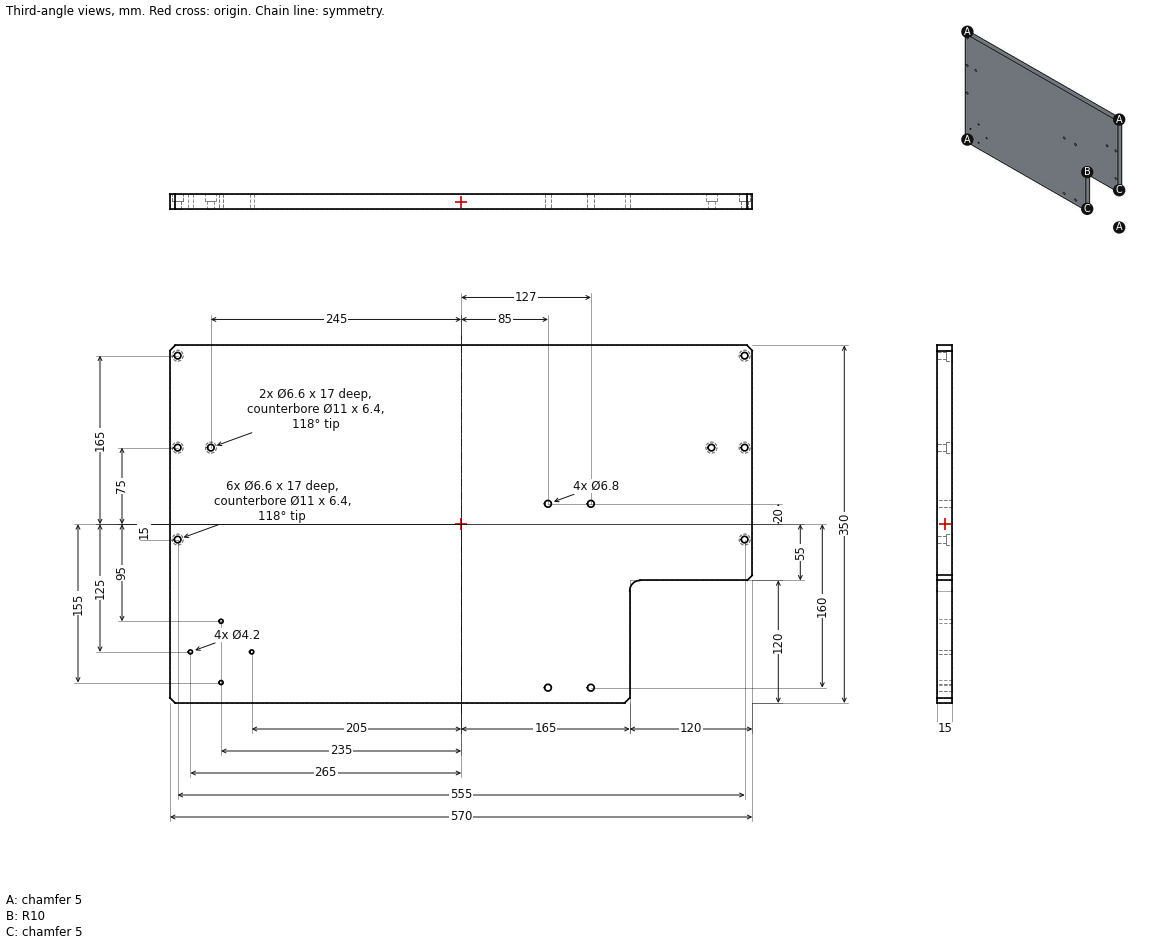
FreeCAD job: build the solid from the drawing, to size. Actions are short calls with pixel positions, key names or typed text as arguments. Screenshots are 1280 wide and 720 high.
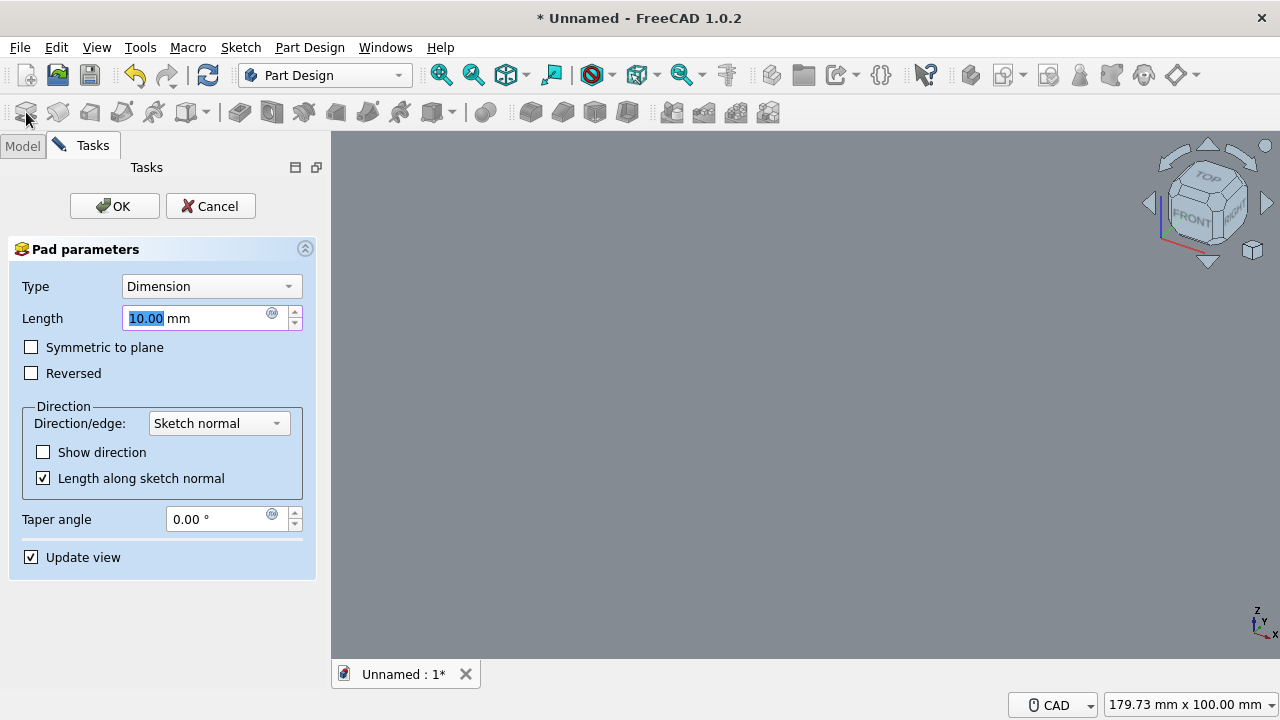
text(15)
key(Tab)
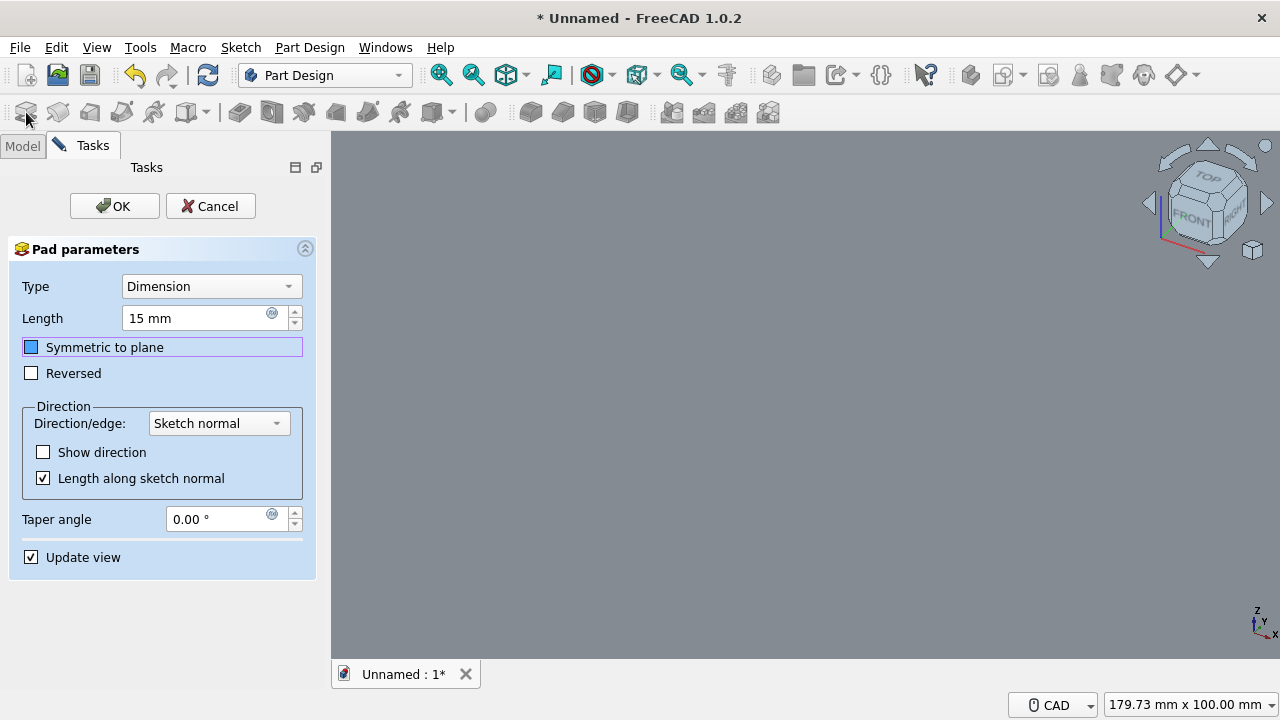
click(30, 347)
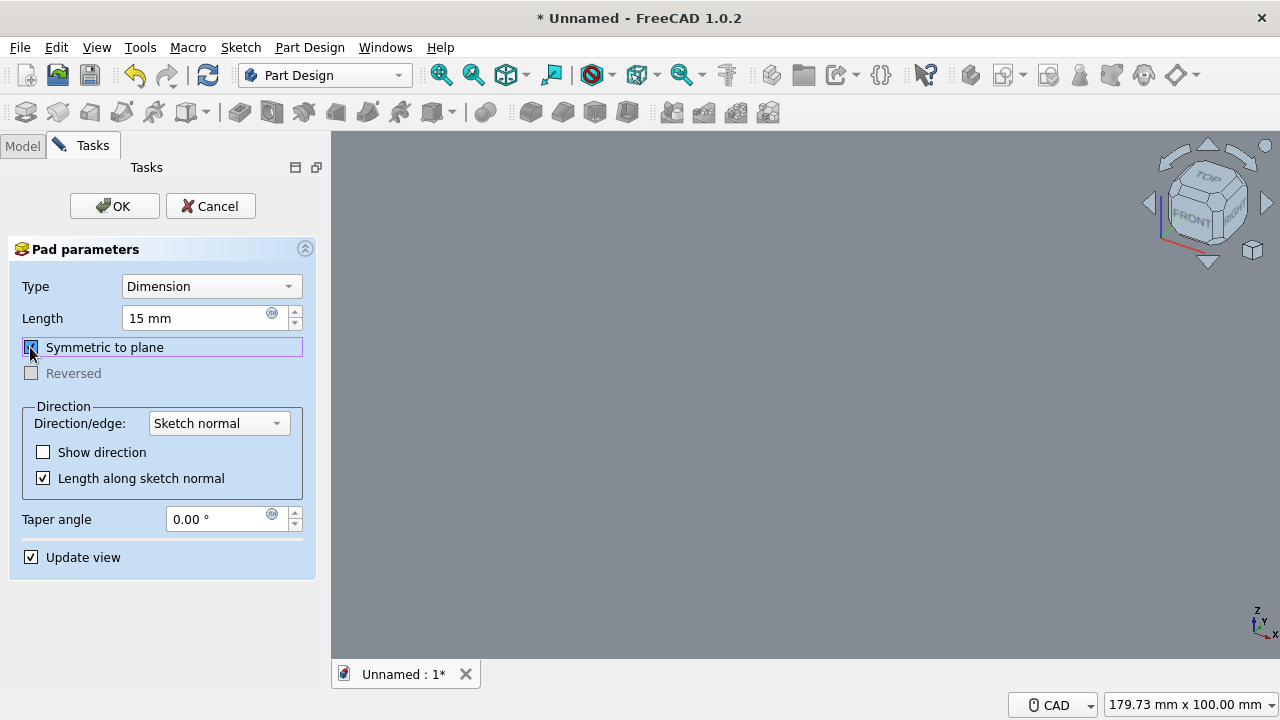
click(115, 206)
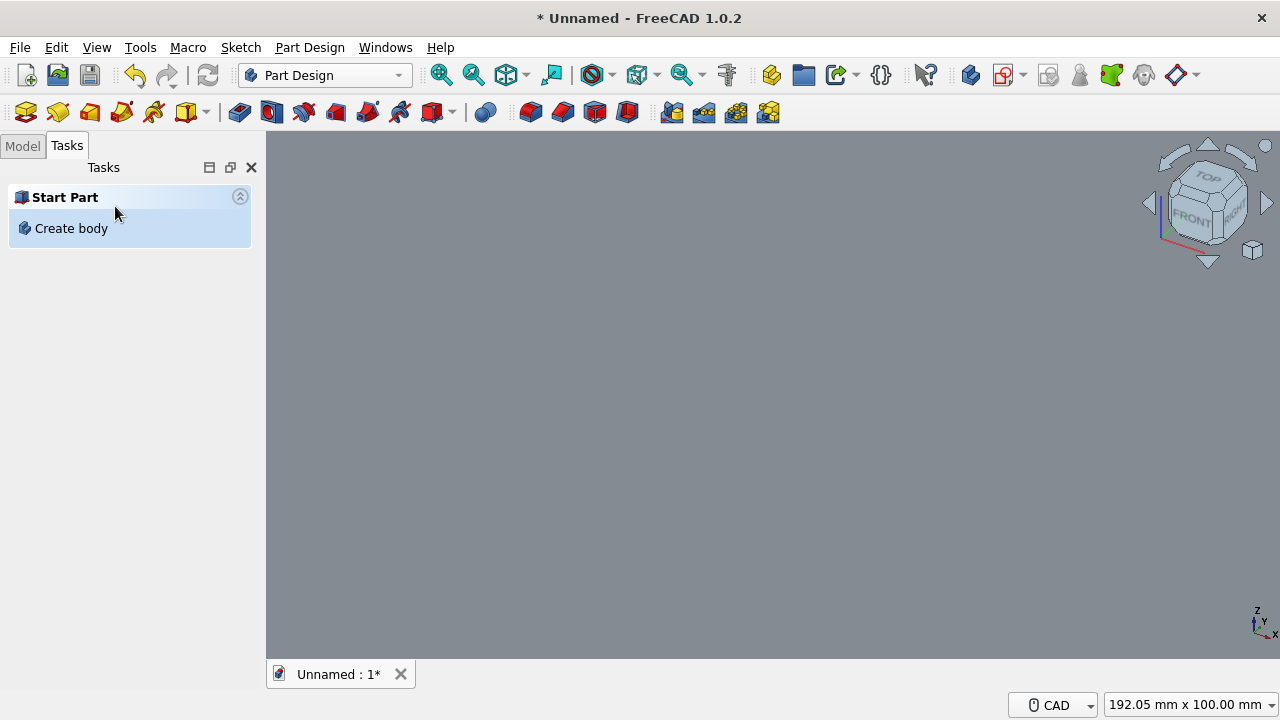
click(442, 76)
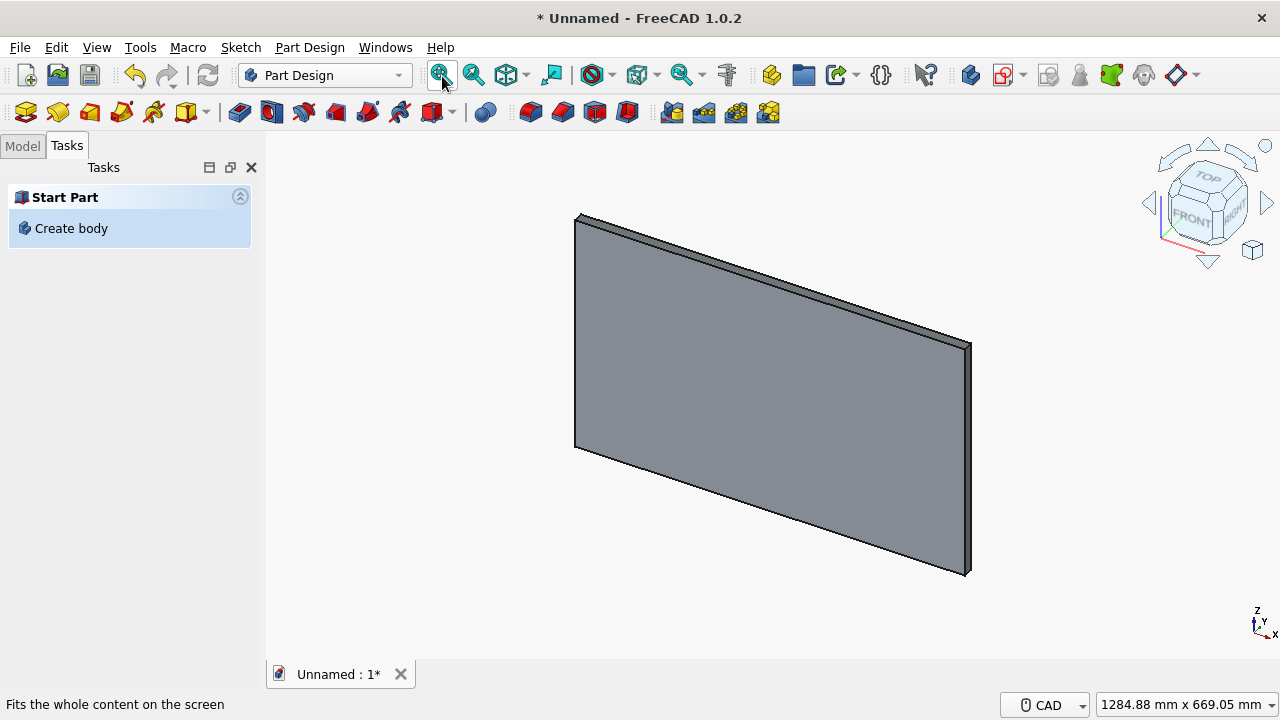
click(970, 344)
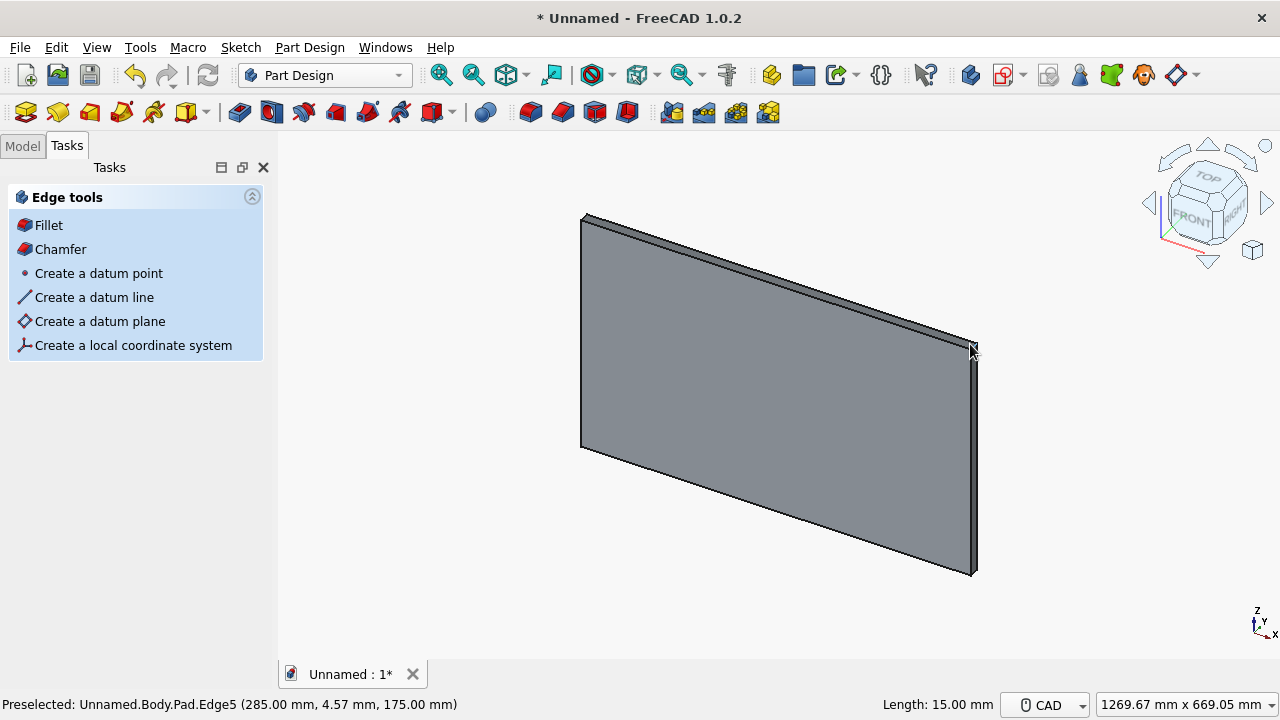
scroll(584, 443, up, 7)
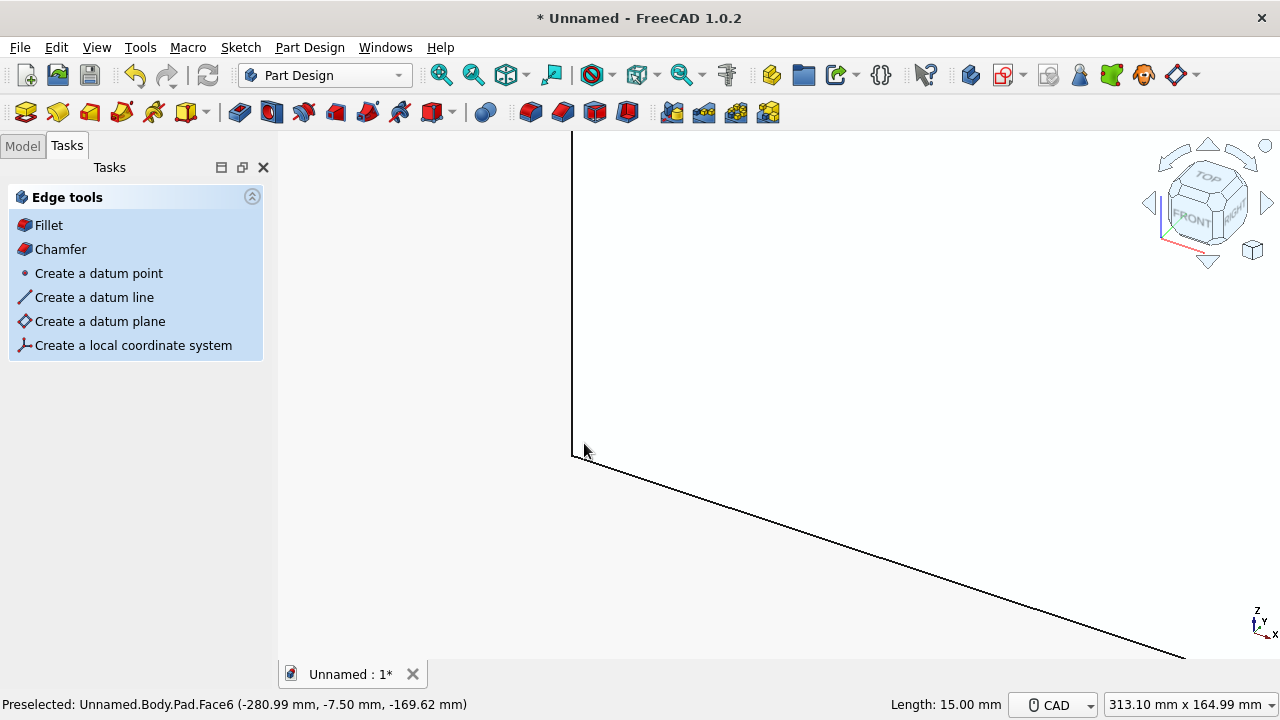
click(442, 76)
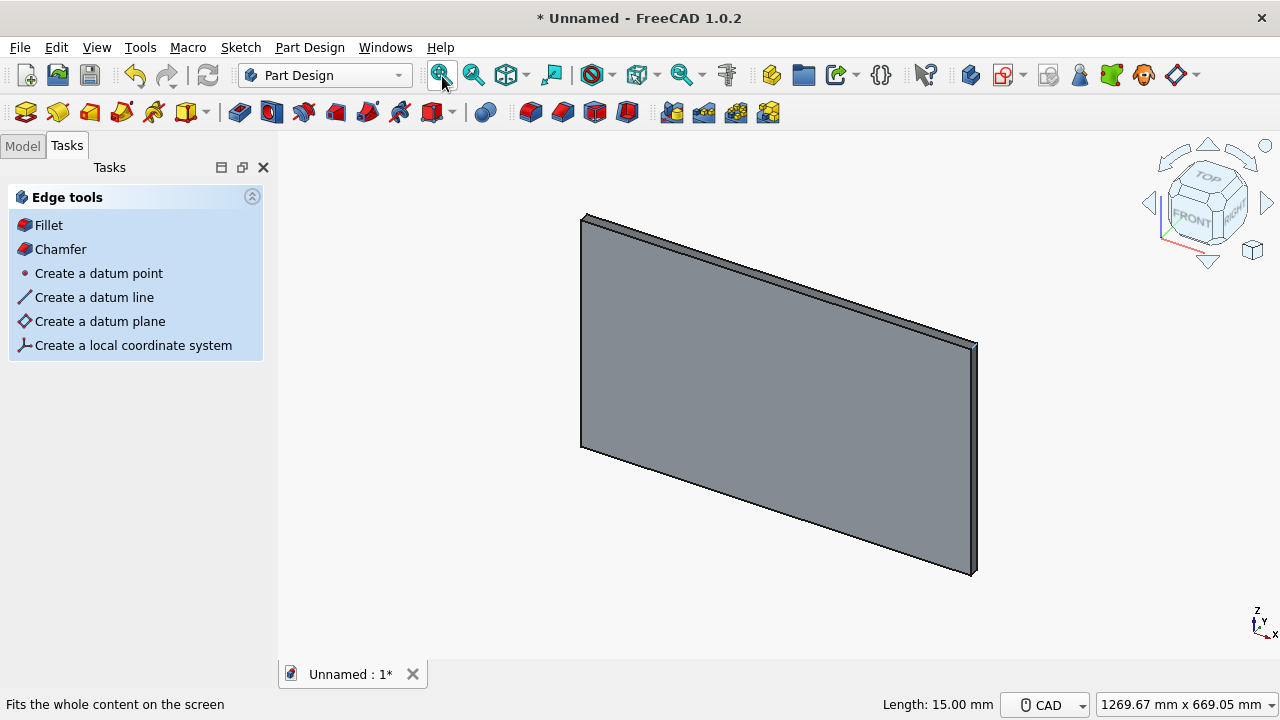
key(0)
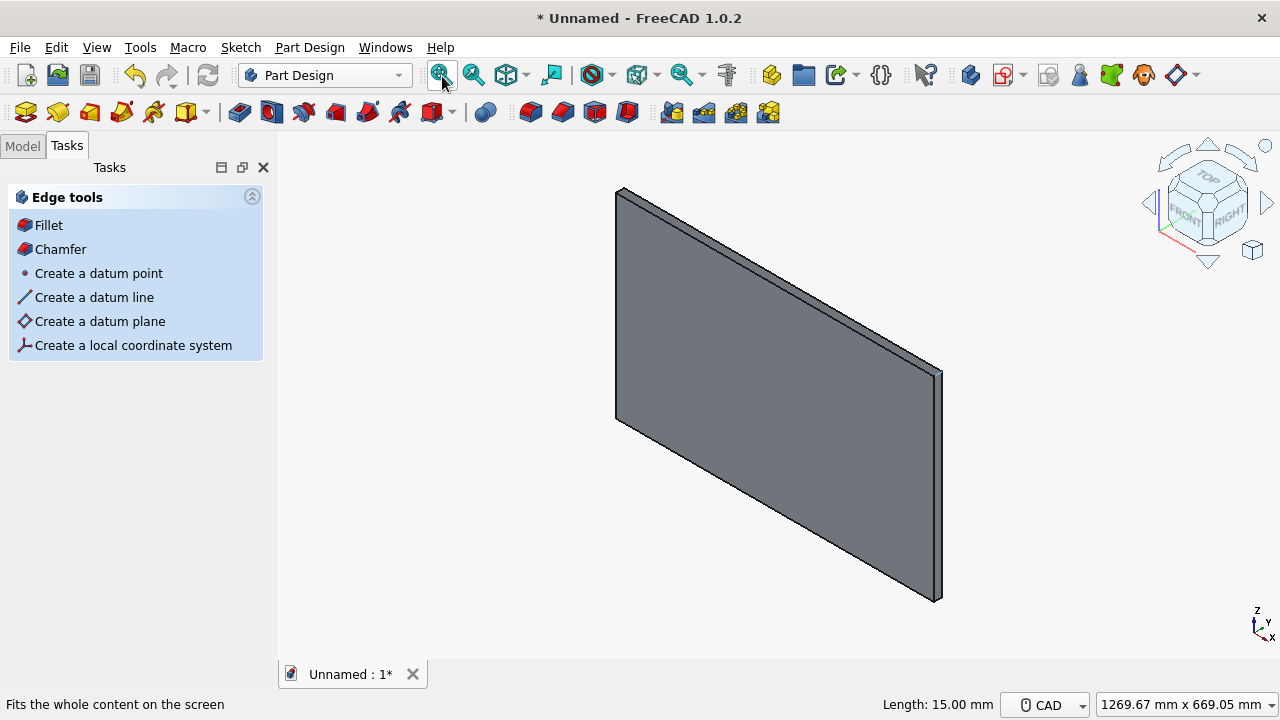
scroll(620, 415, up, 7)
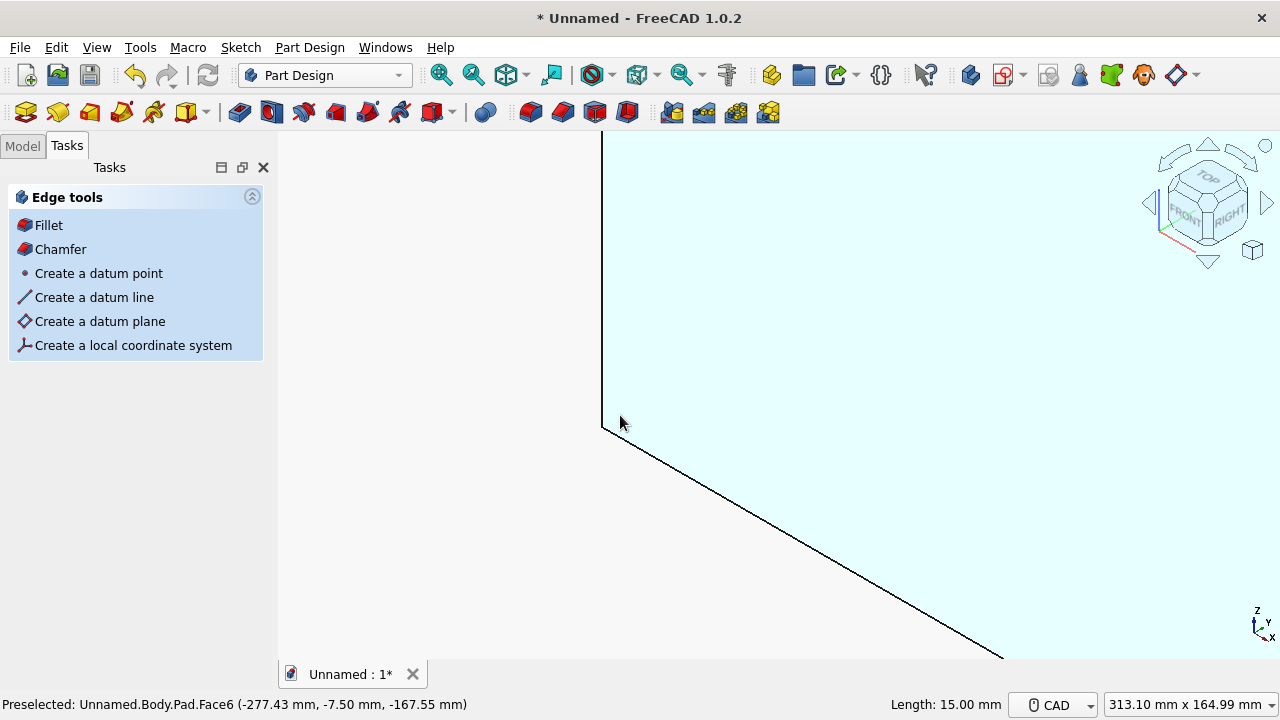
click(442, 76)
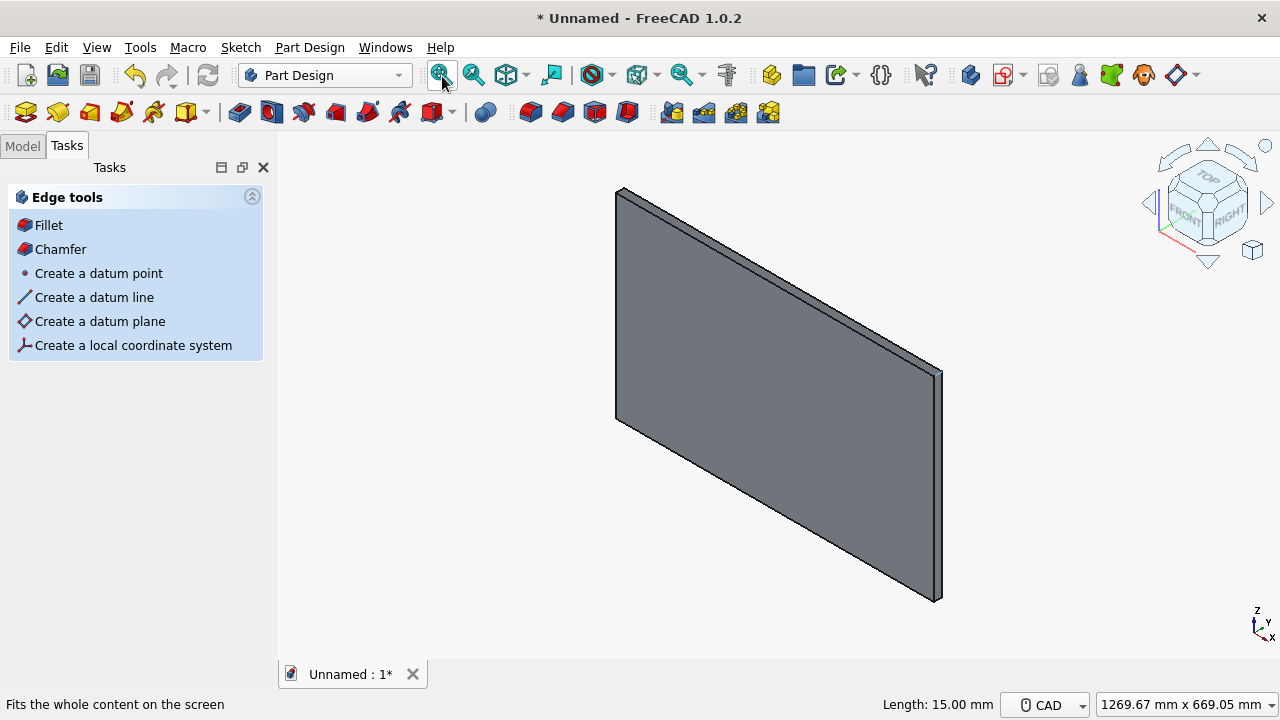
key(2)